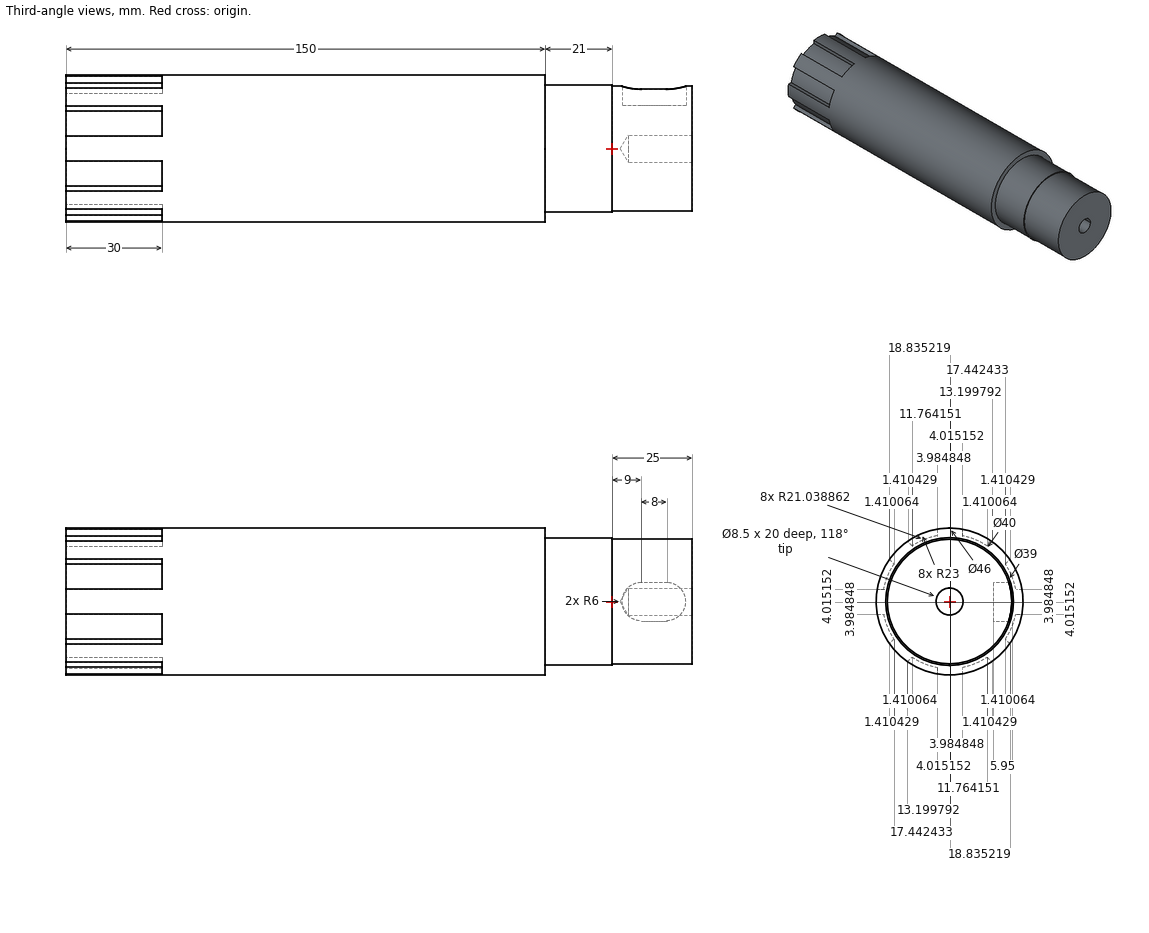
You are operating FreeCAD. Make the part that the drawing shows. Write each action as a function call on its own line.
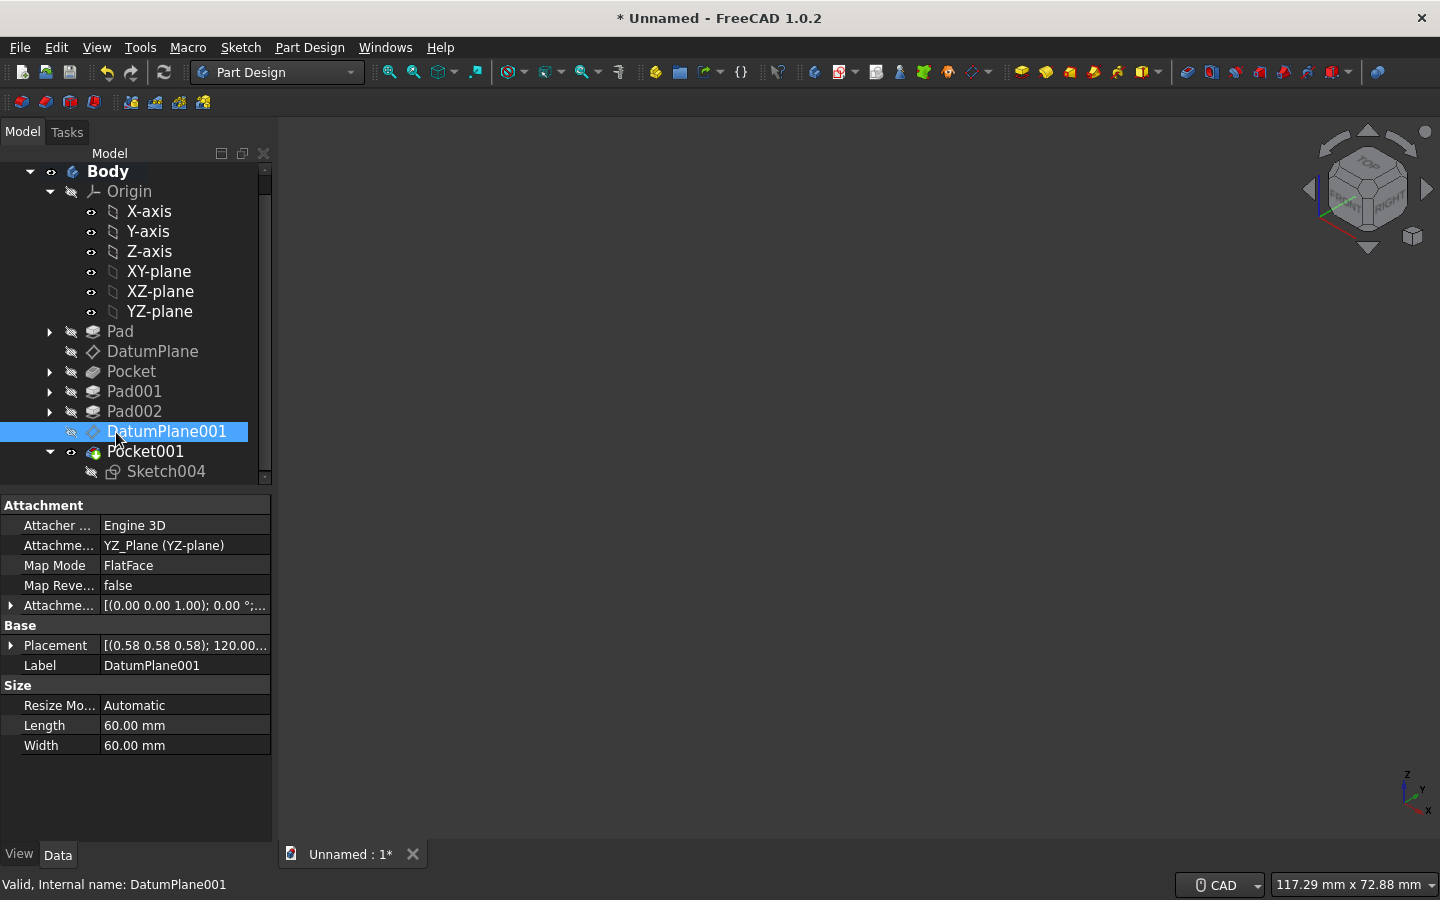
click(390, 72)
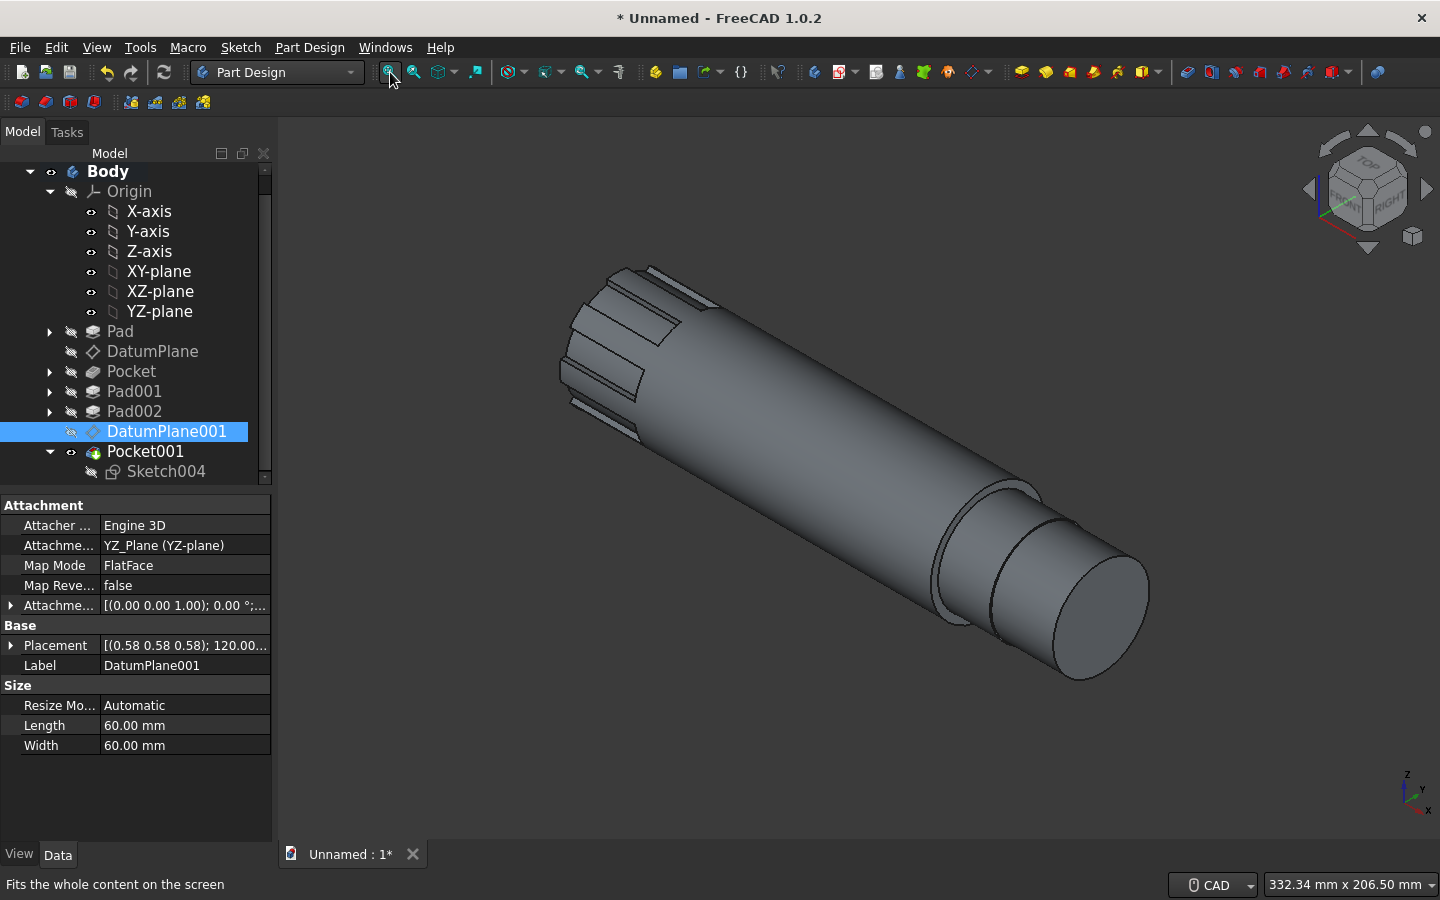
click(1101, 617)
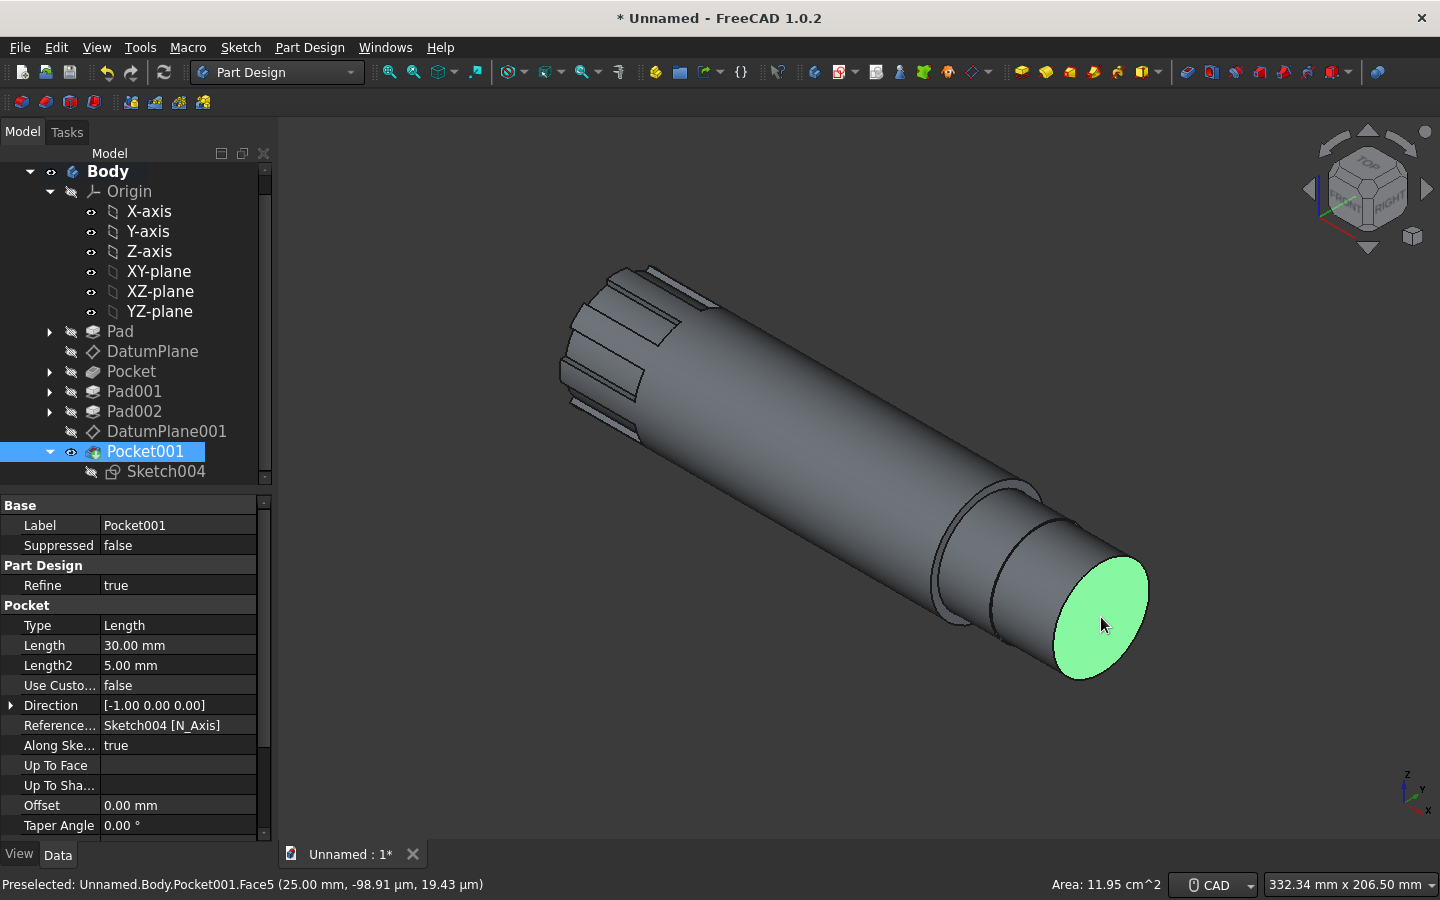
click(840, 72)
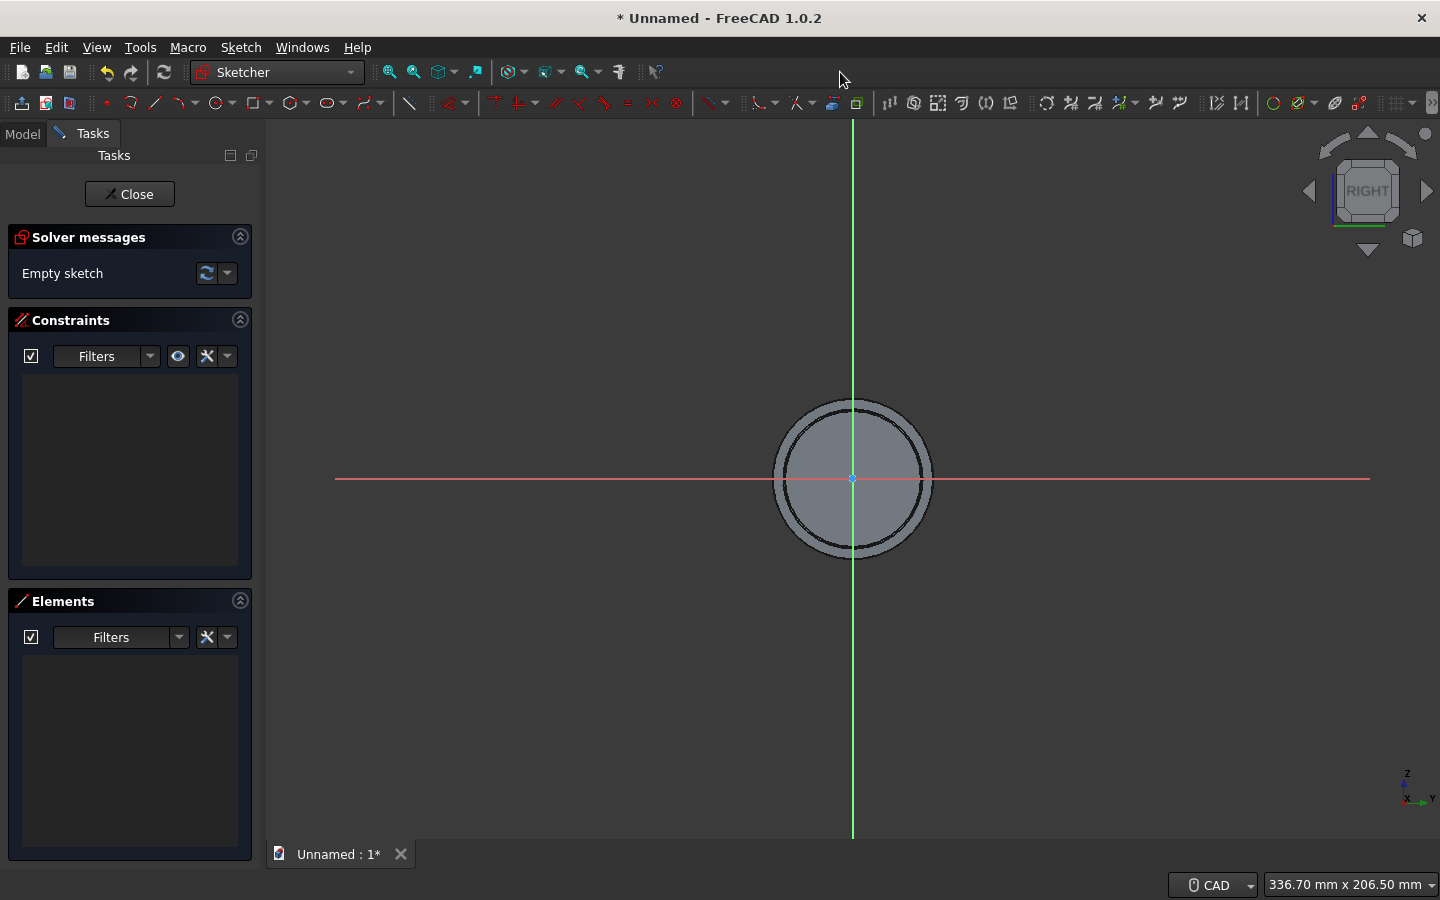
scroll(857, 479, up, 14)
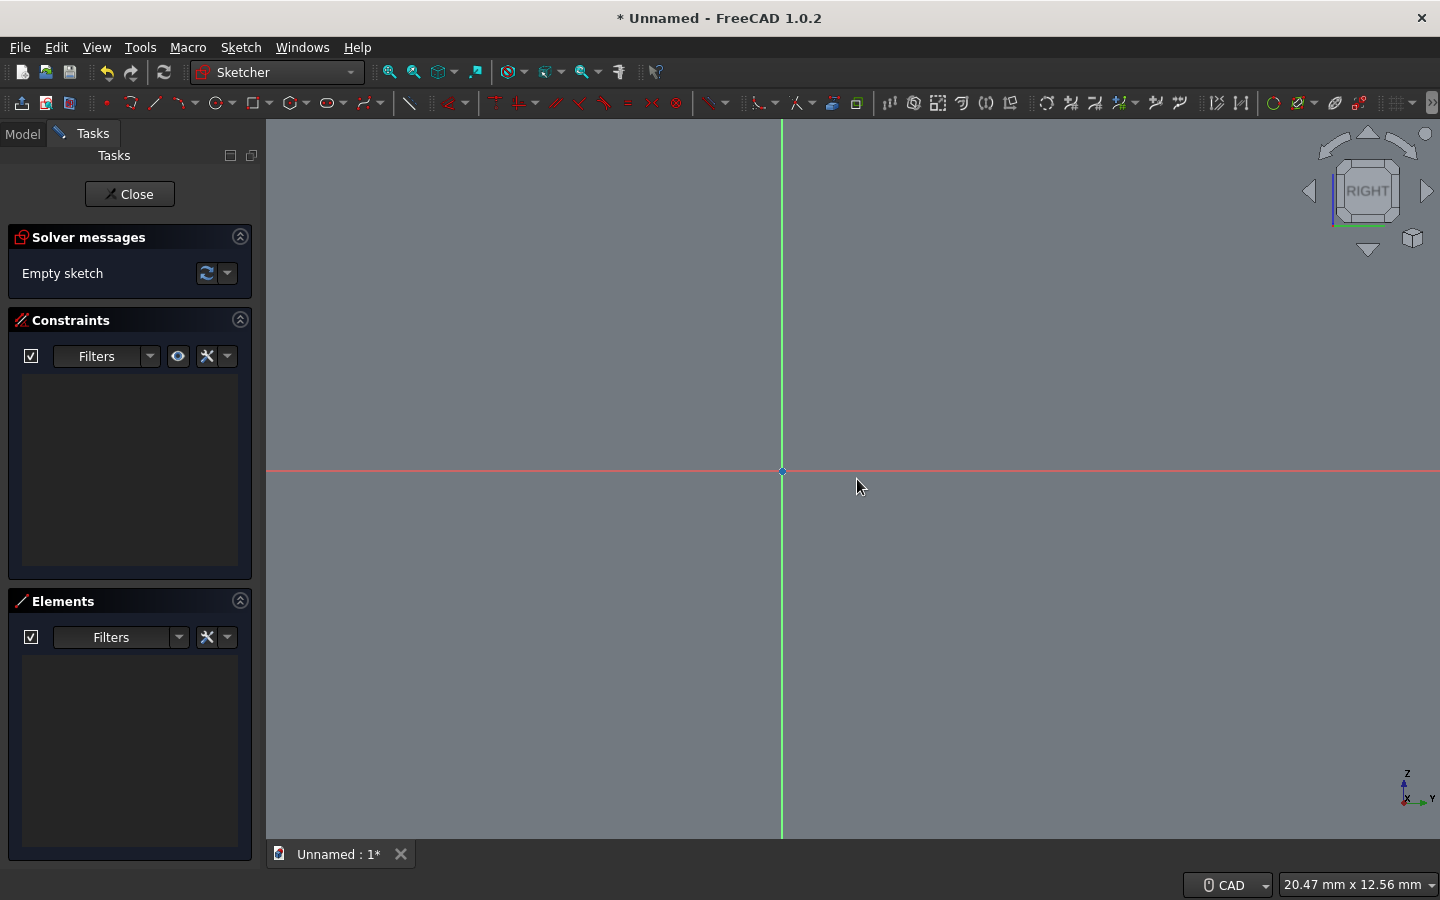
click(216, 104)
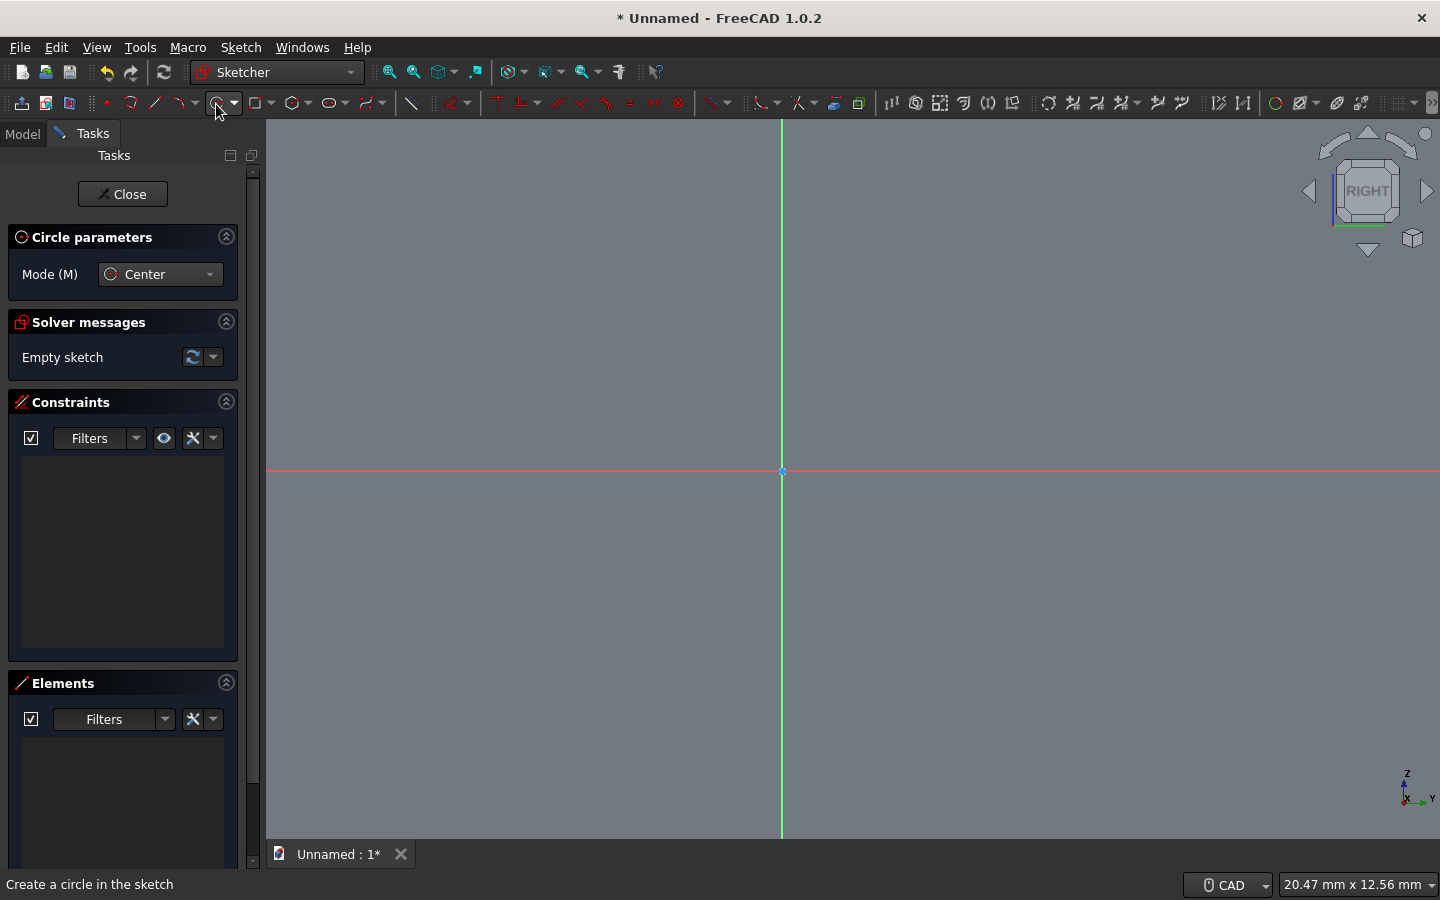
click(782, 471)
click(955, 299)
key(Escape)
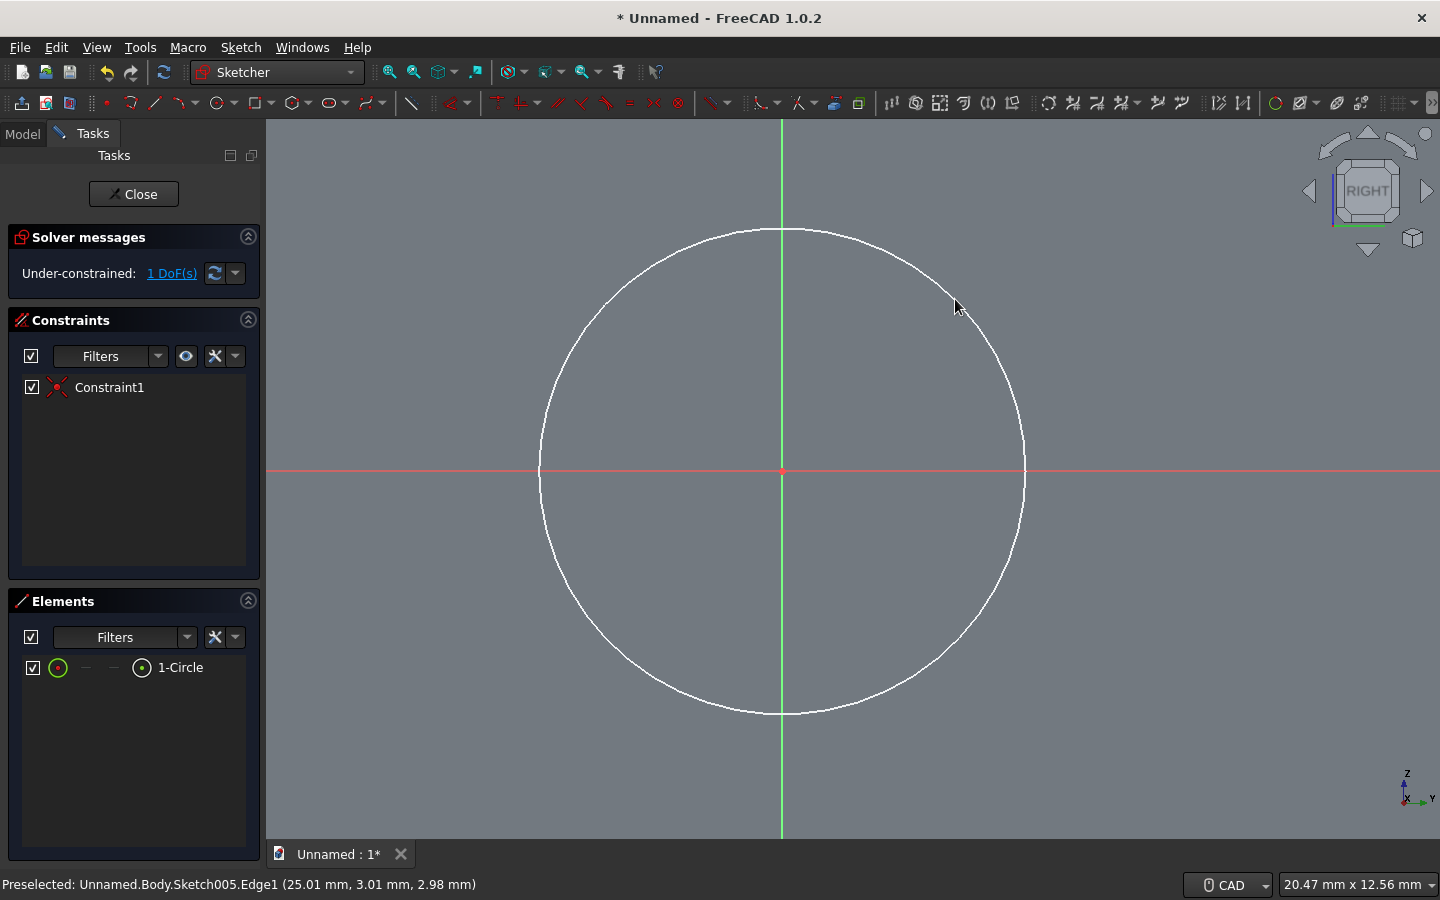
click(450, 104)